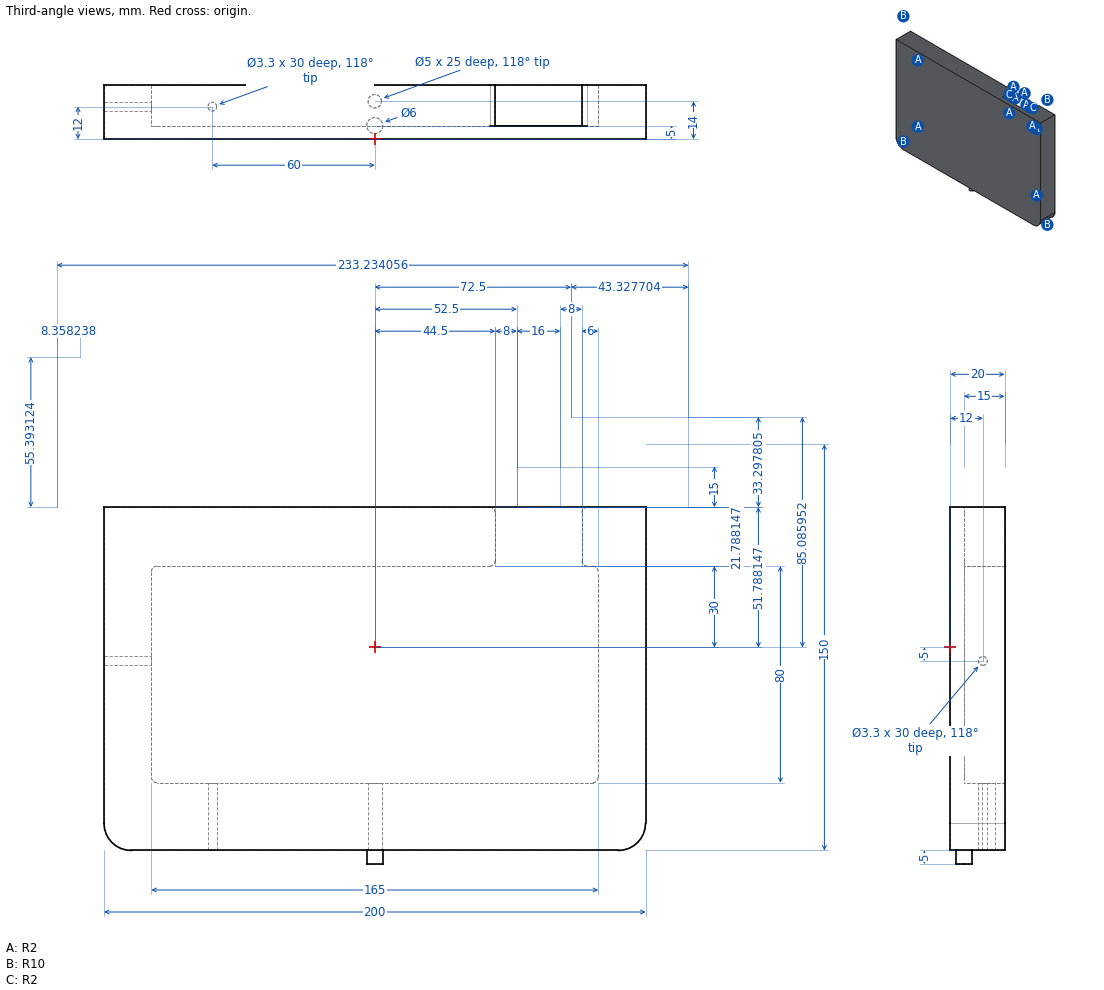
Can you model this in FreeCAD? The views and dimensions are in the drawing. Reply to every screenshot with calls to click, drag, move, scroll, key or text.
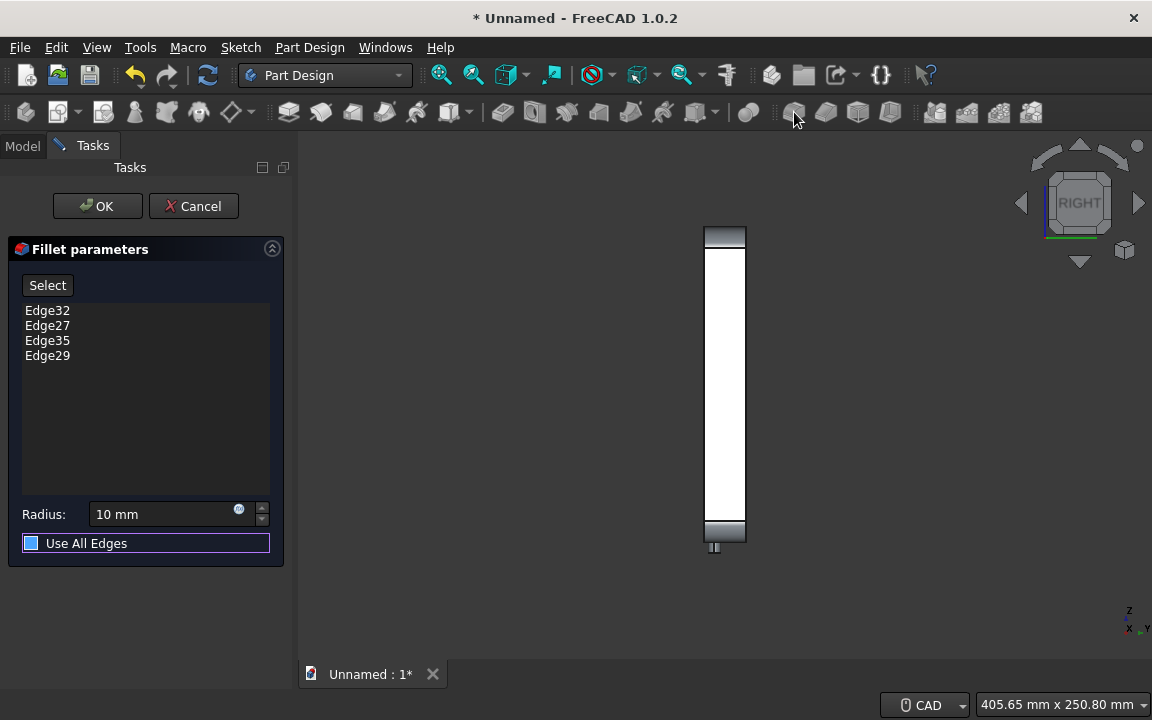
click(98, 206)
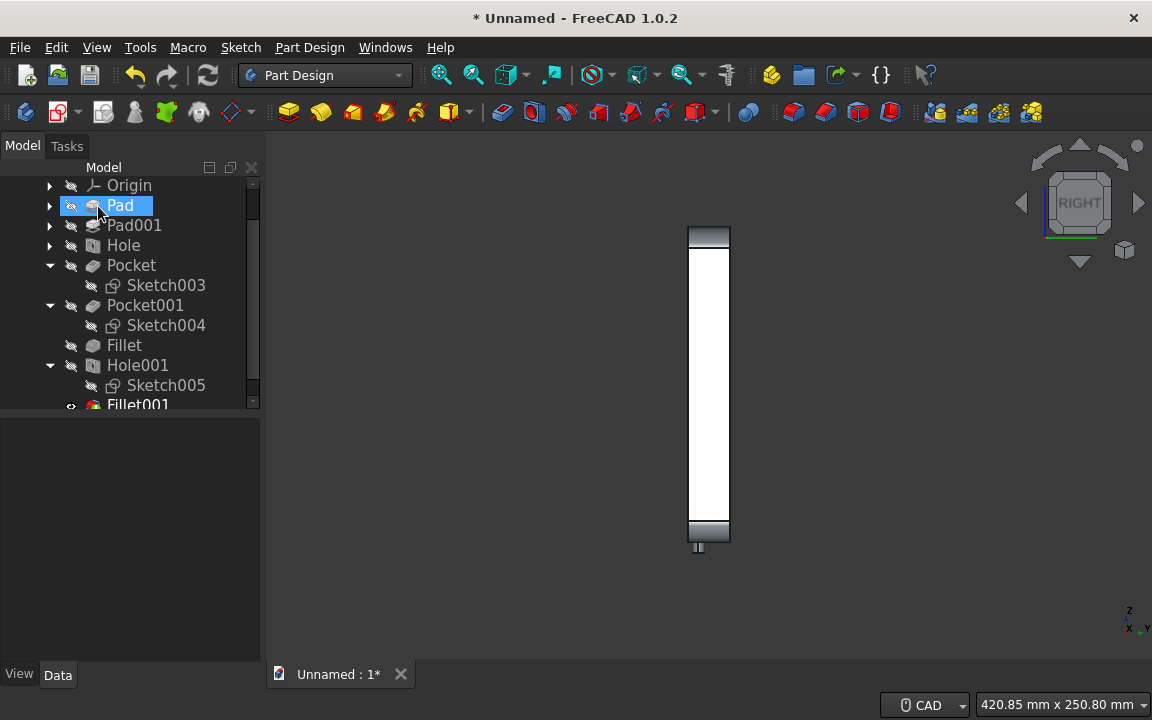
key(5)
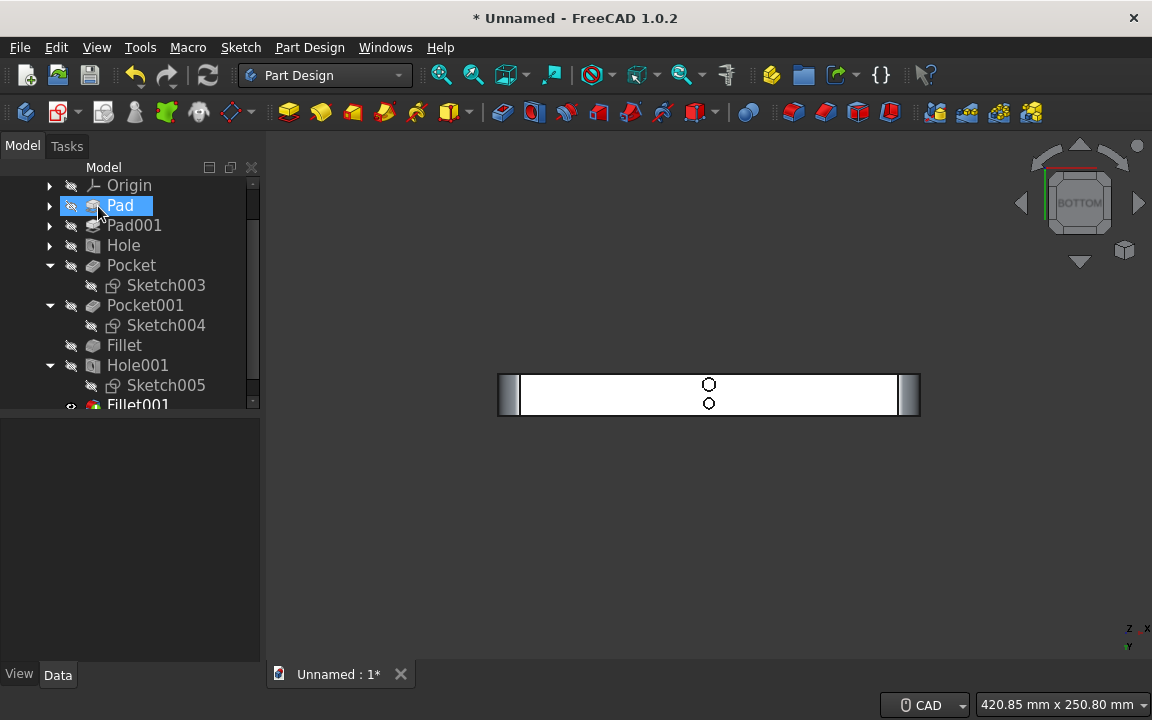
click(871, 394)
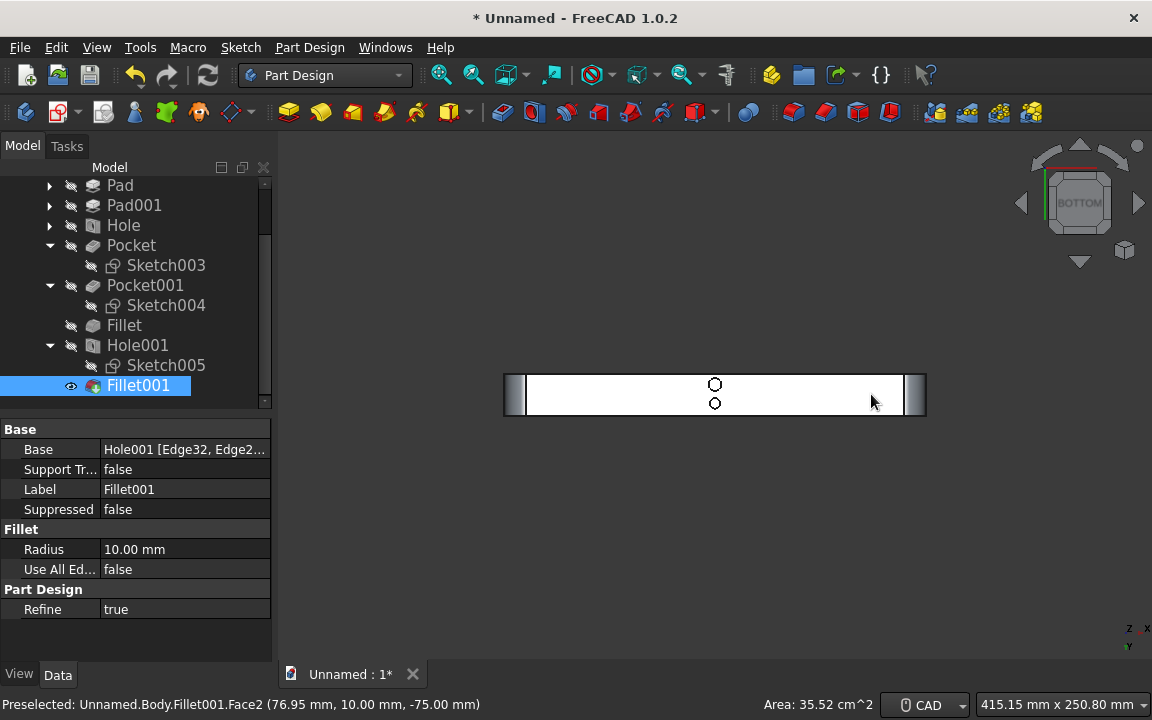
click(58, 112)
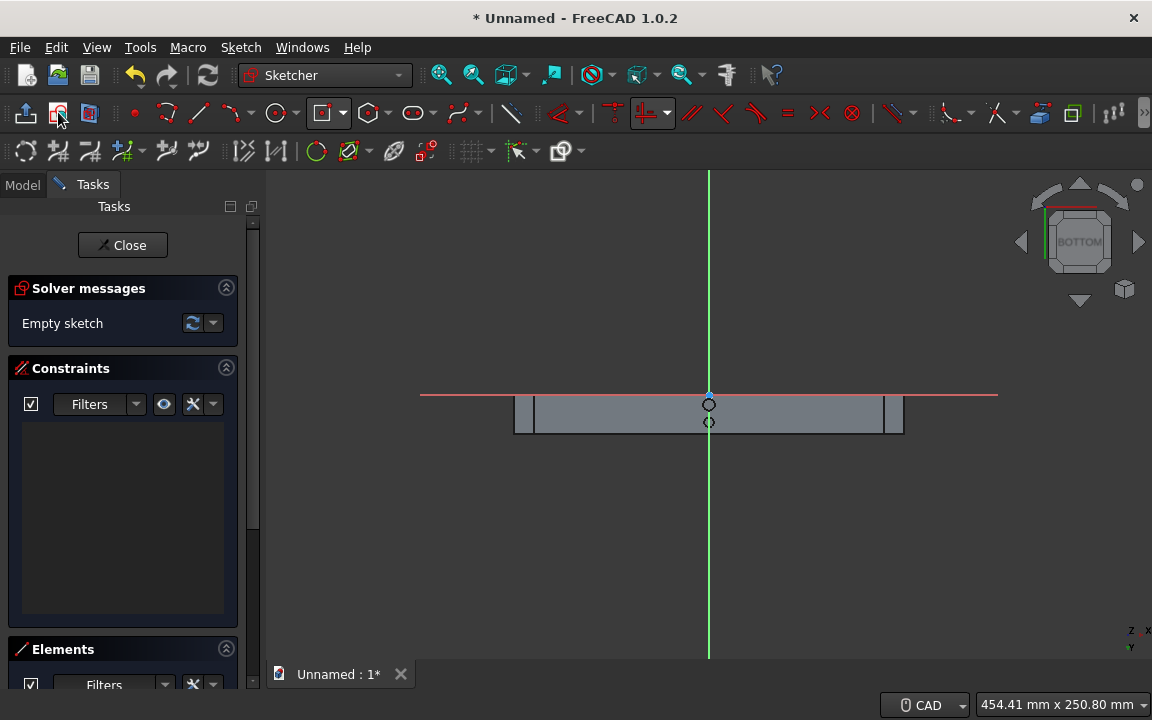
key(q)
key(s)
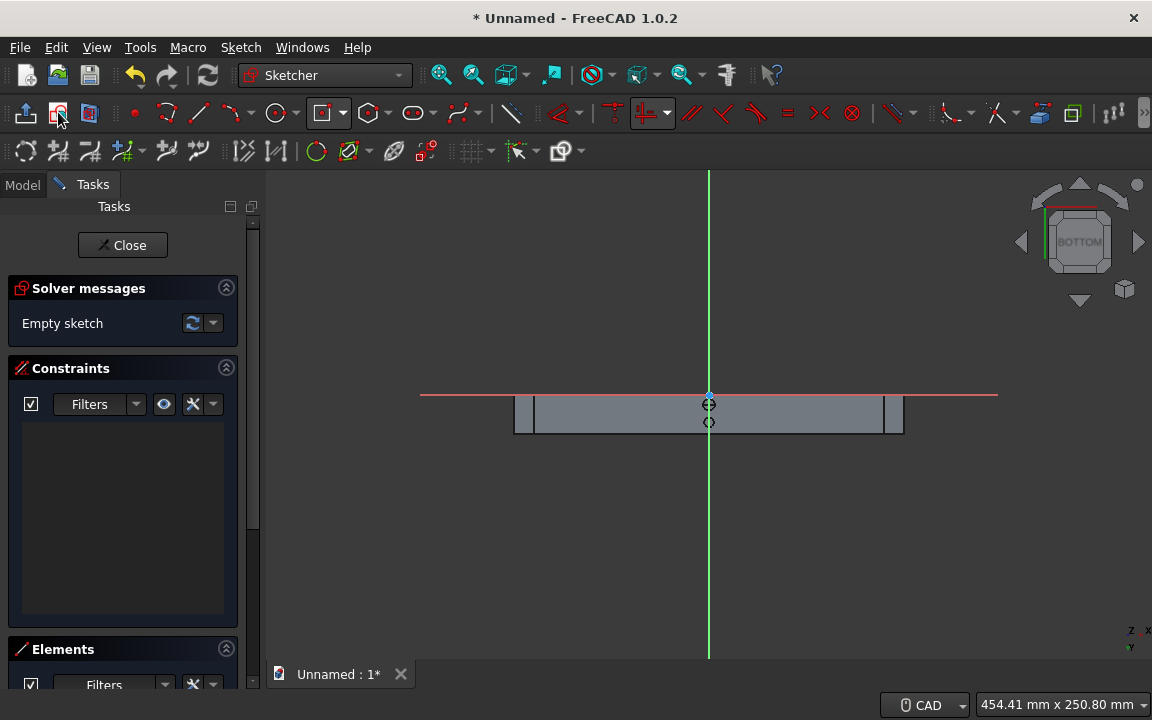
scroll(589, 419, up, 15)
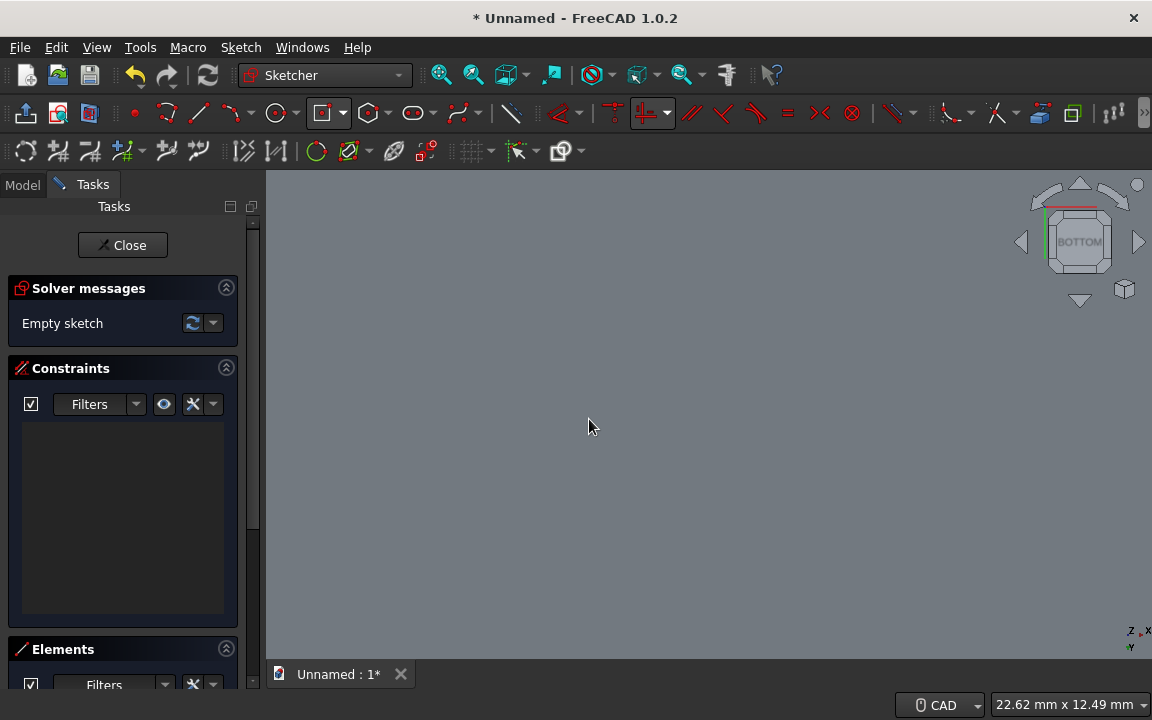
scroll(644, 383, up, 4)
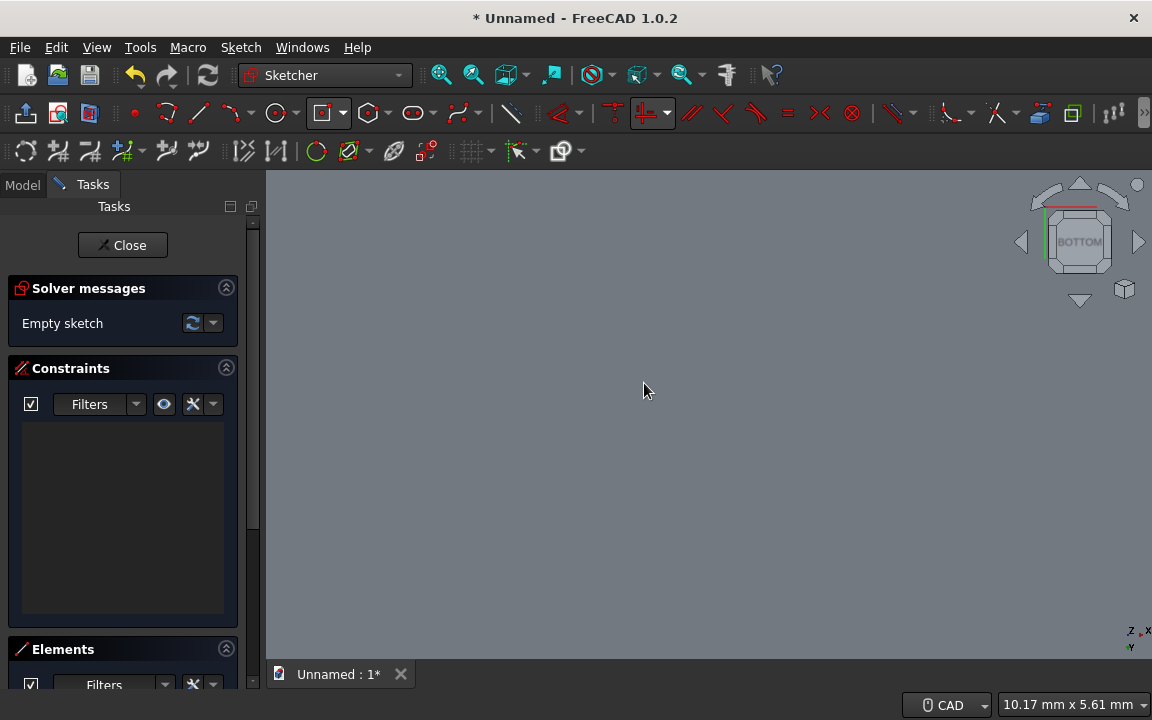
key(g)
key(c)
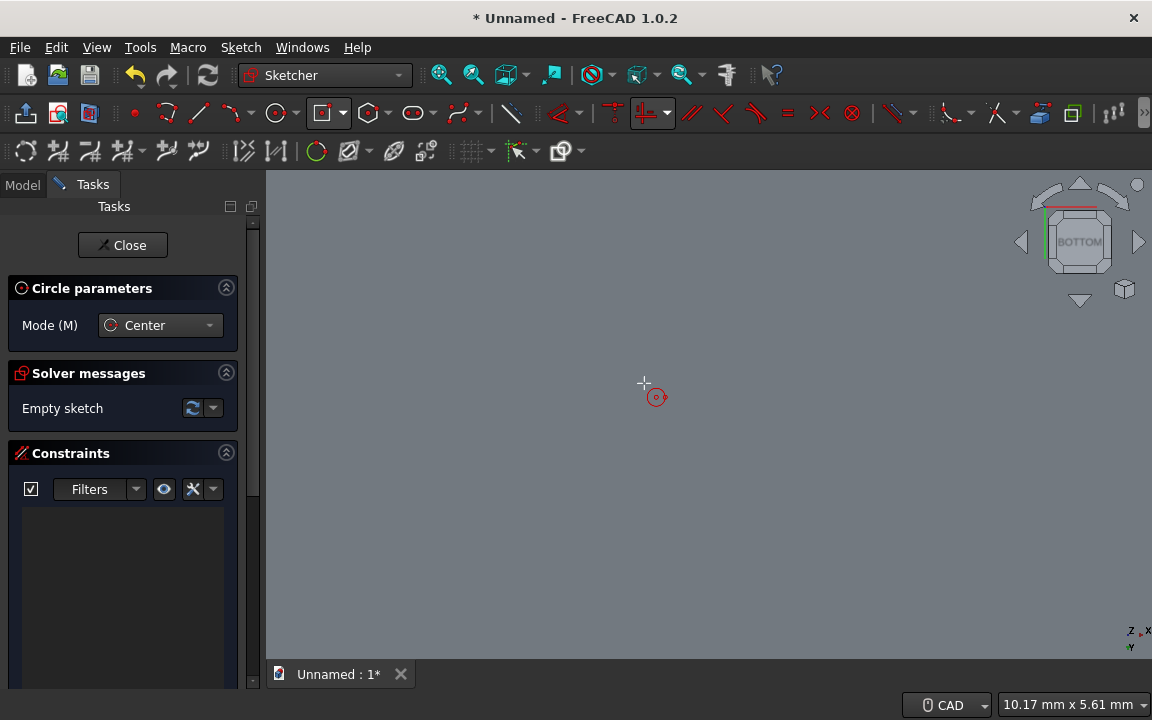
click(640, 414)
click(742, 312)
key(Escape)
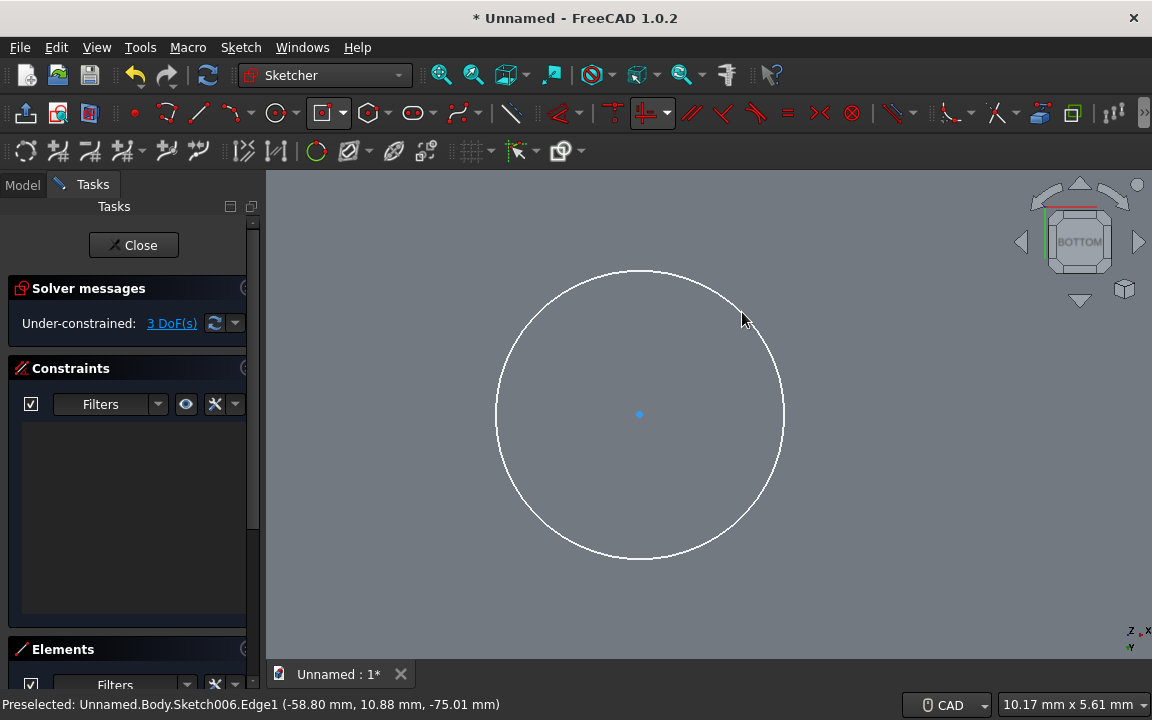
key(d)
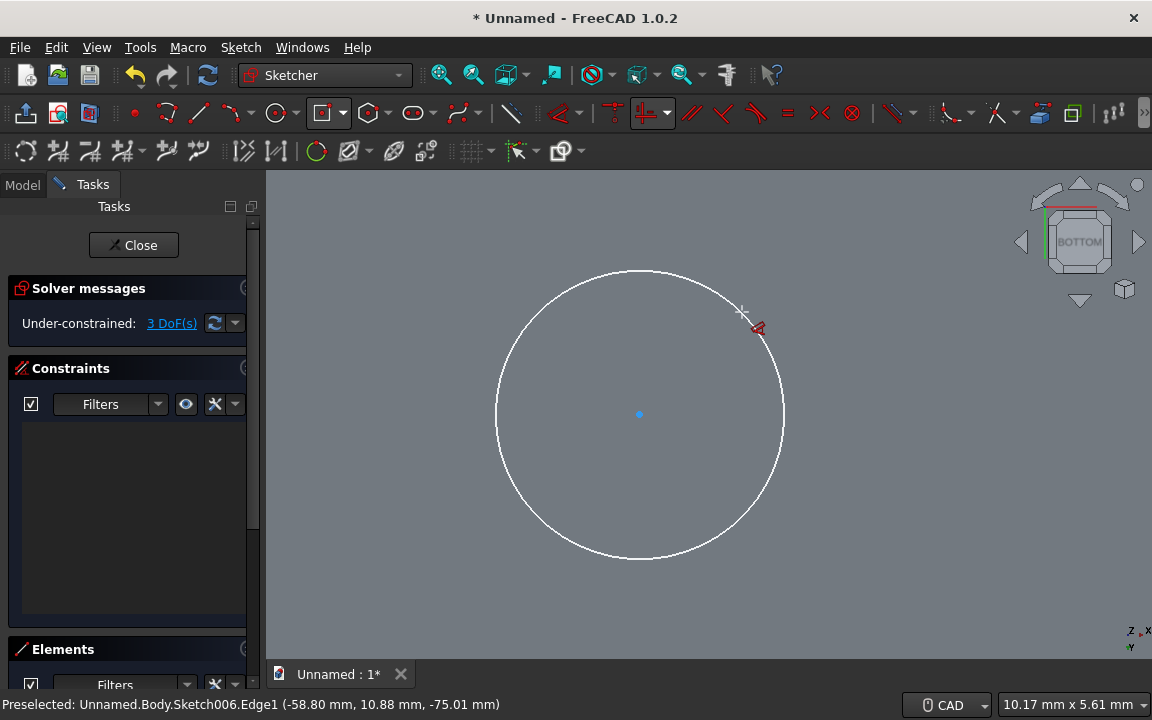
click(742, 313)
click(765, 290)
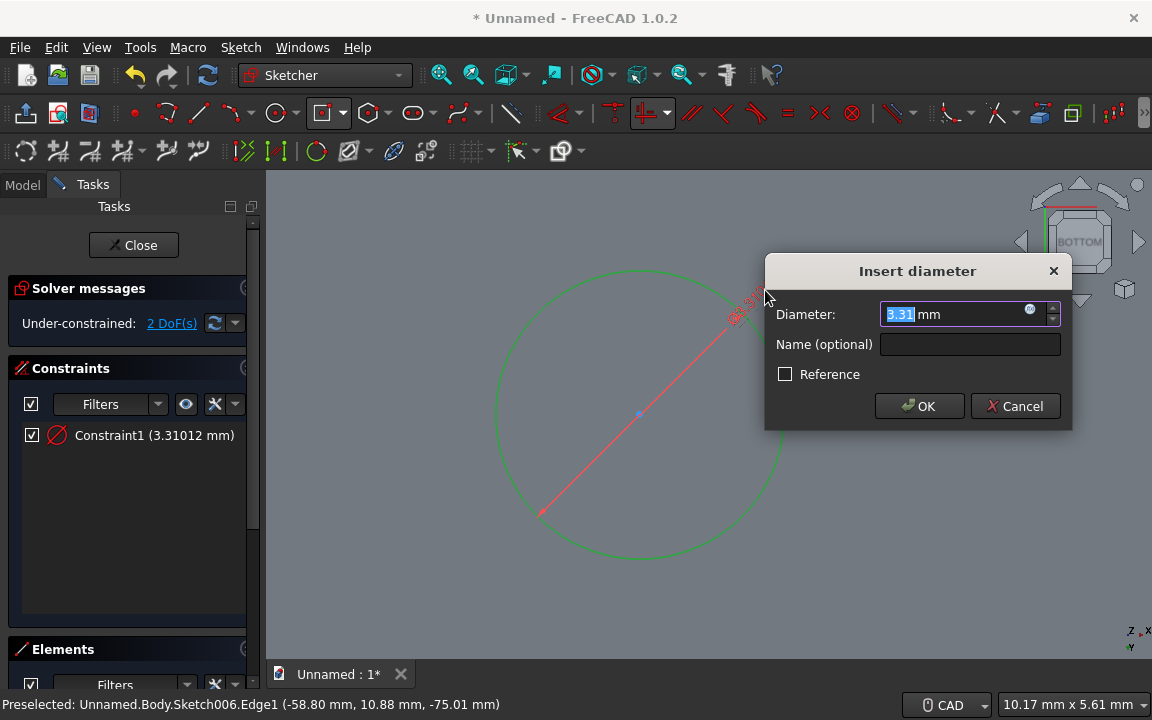
text(3.3)
key(Return)